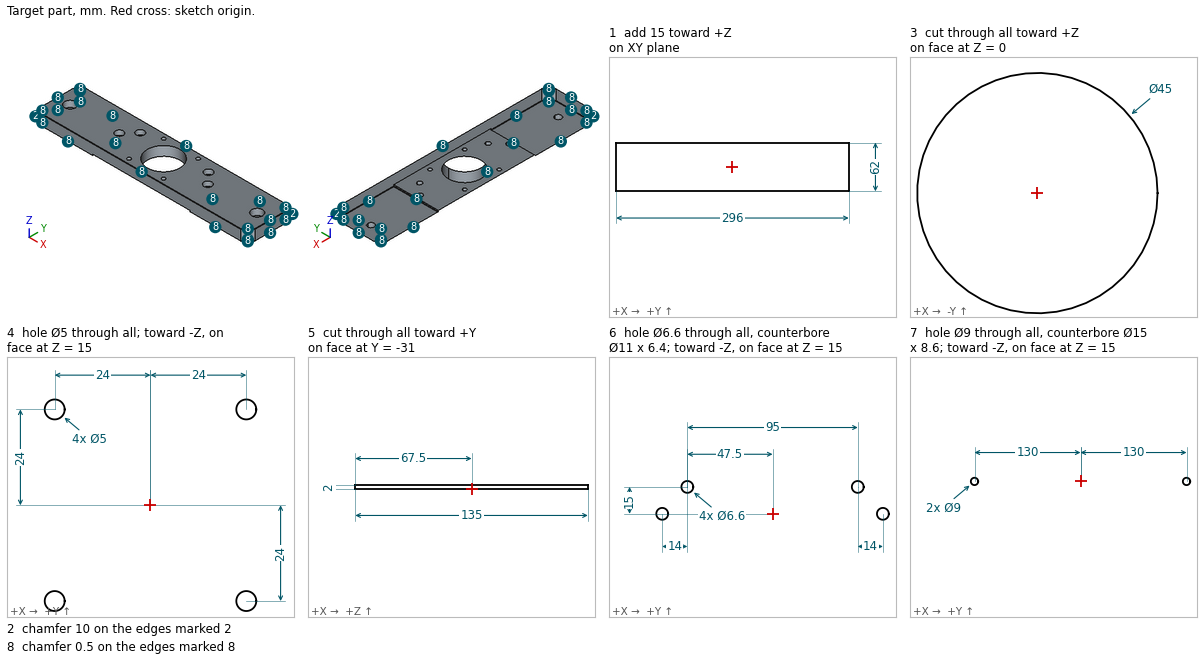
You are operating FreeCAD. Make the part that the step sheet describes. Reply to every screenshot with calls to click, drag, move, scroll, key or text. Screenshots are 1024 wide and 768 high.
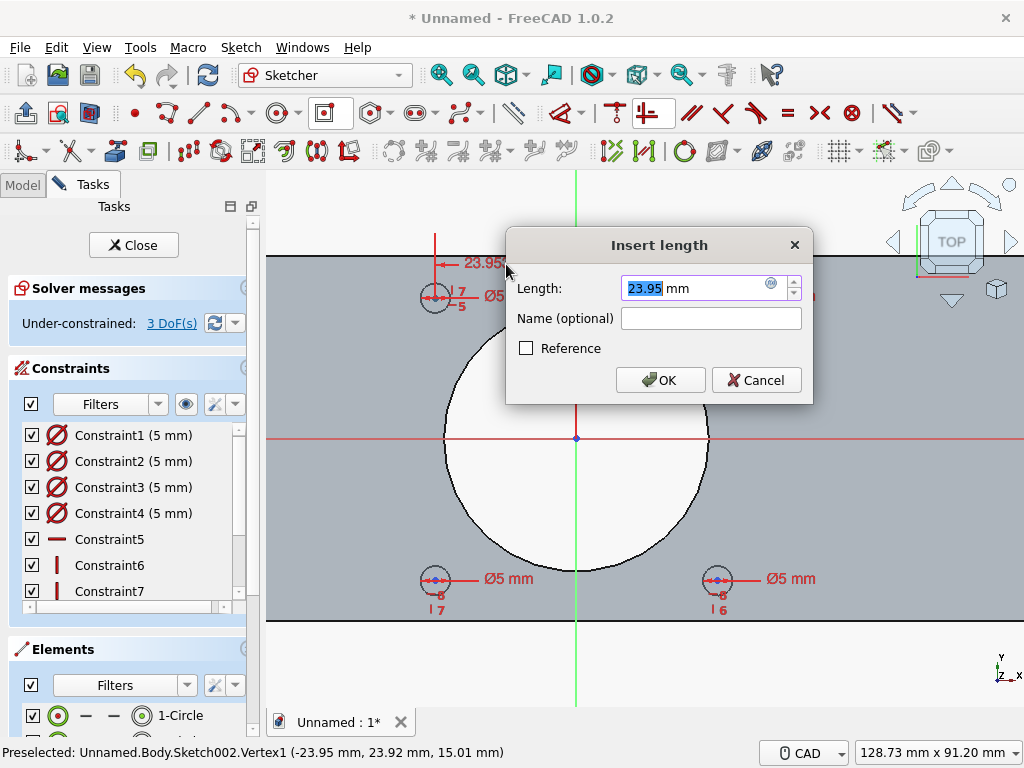
text(24)
key(Return)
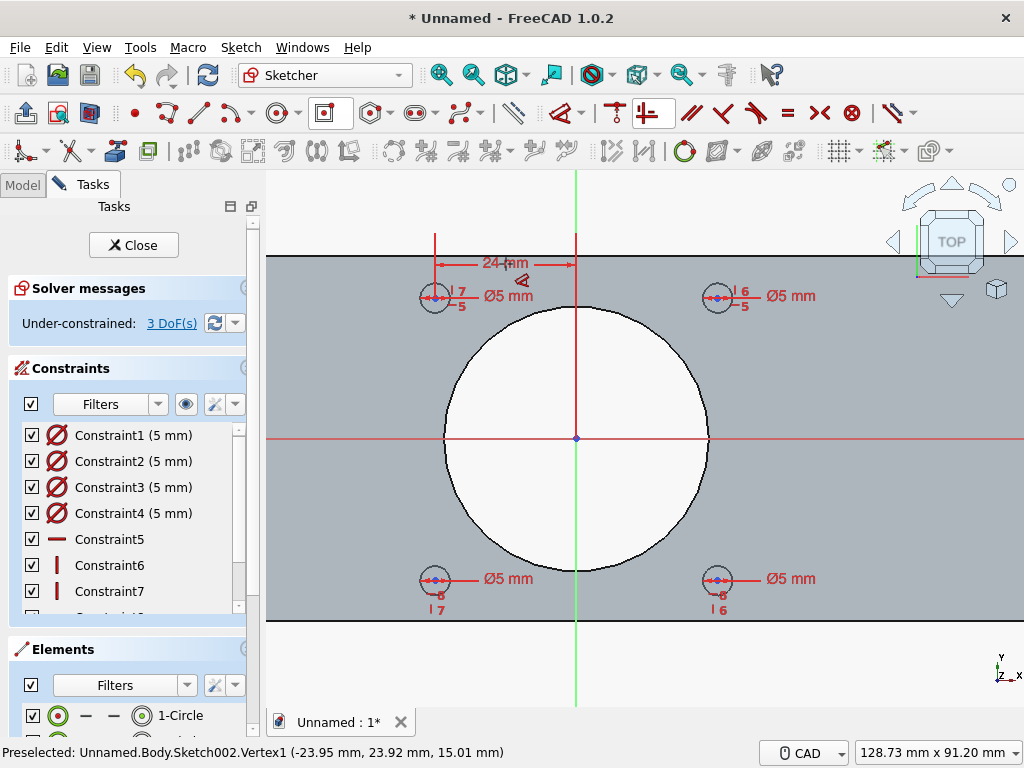
click(435, 298)
click(401, 369)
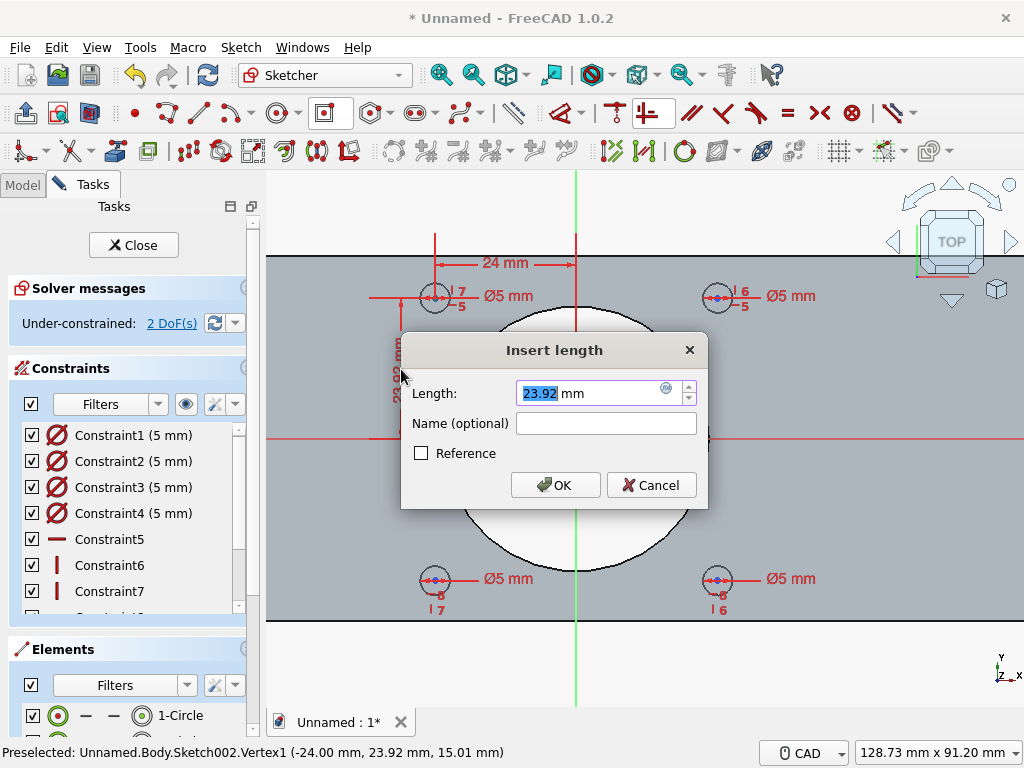
text(24)
key(Return)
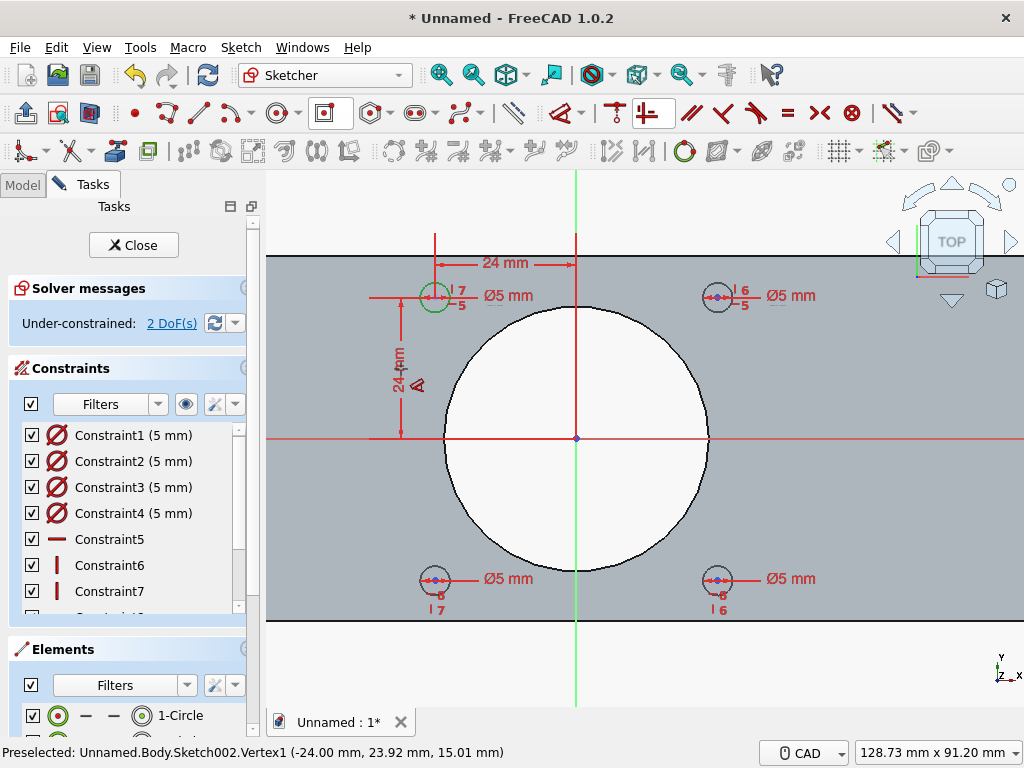
click(718, 298)
click(647, 264)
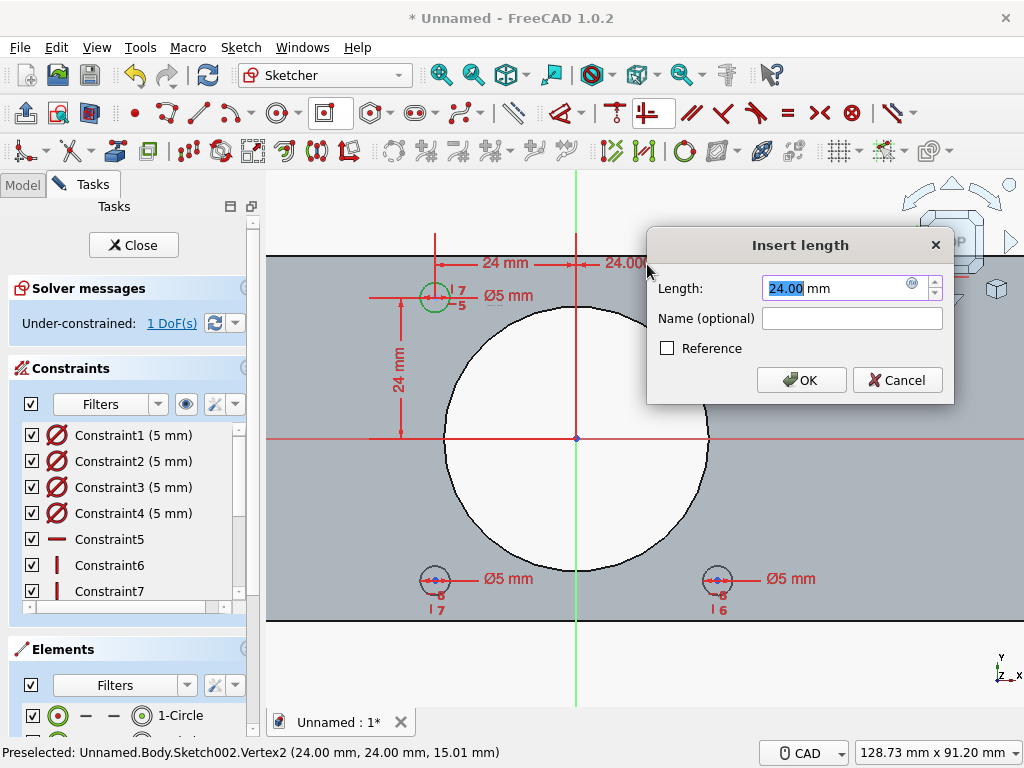
text(24)
key(Return)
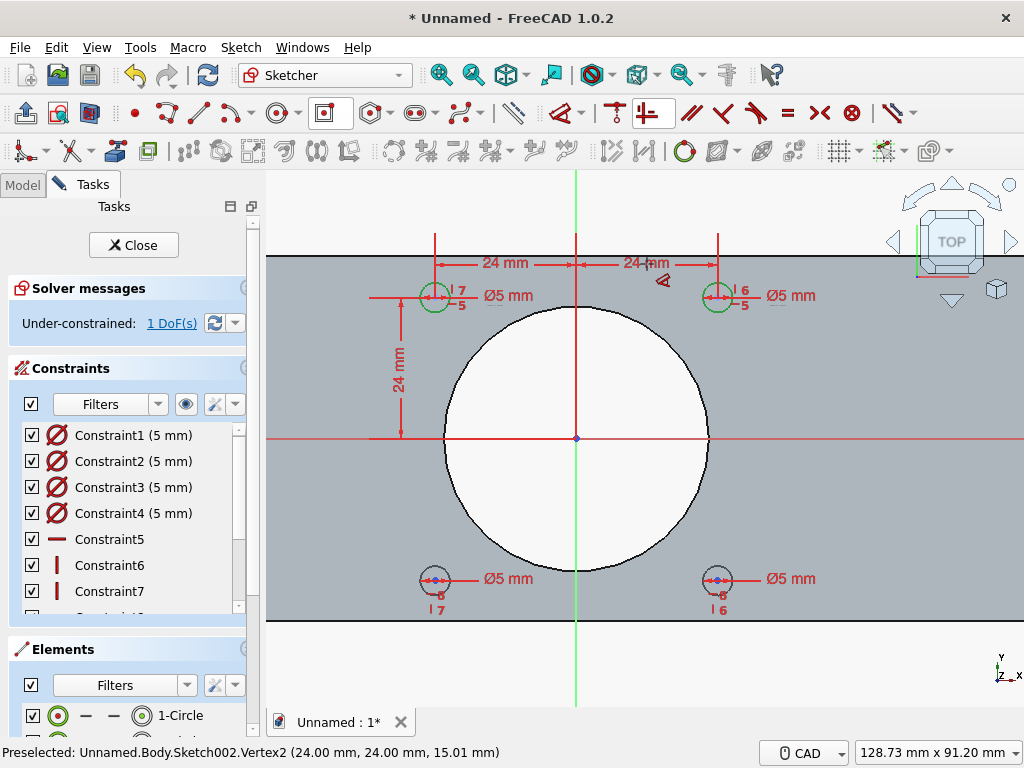
click(718, 581)
click(752, 510)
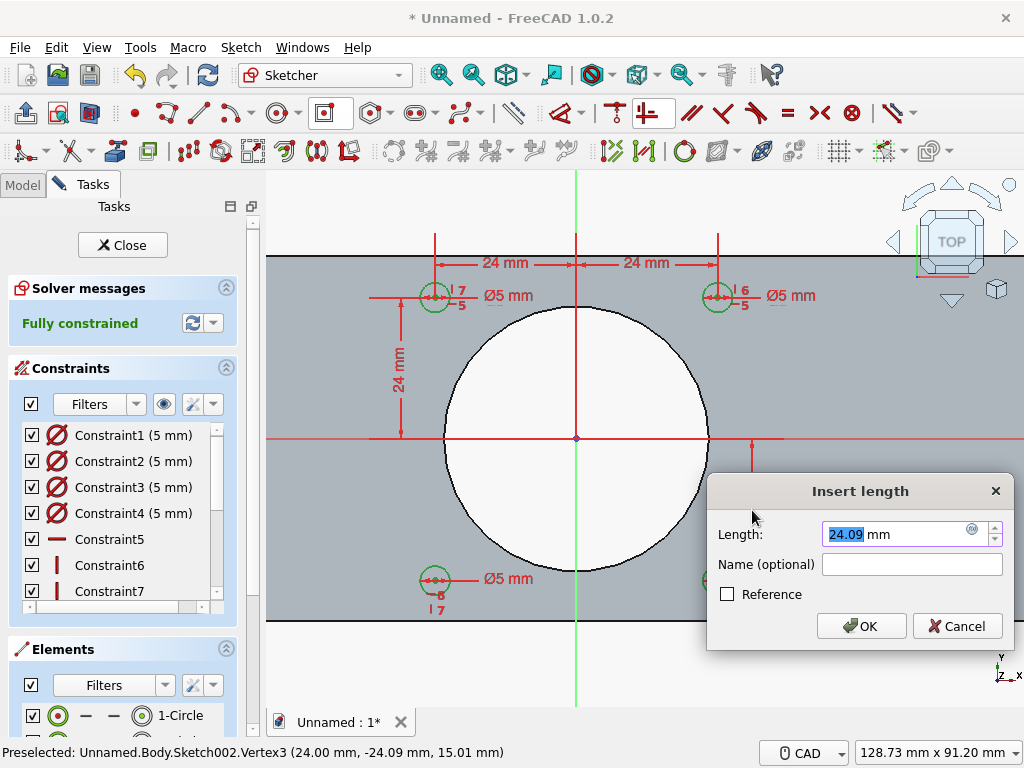
text(24)
key(Return)
key(Escape)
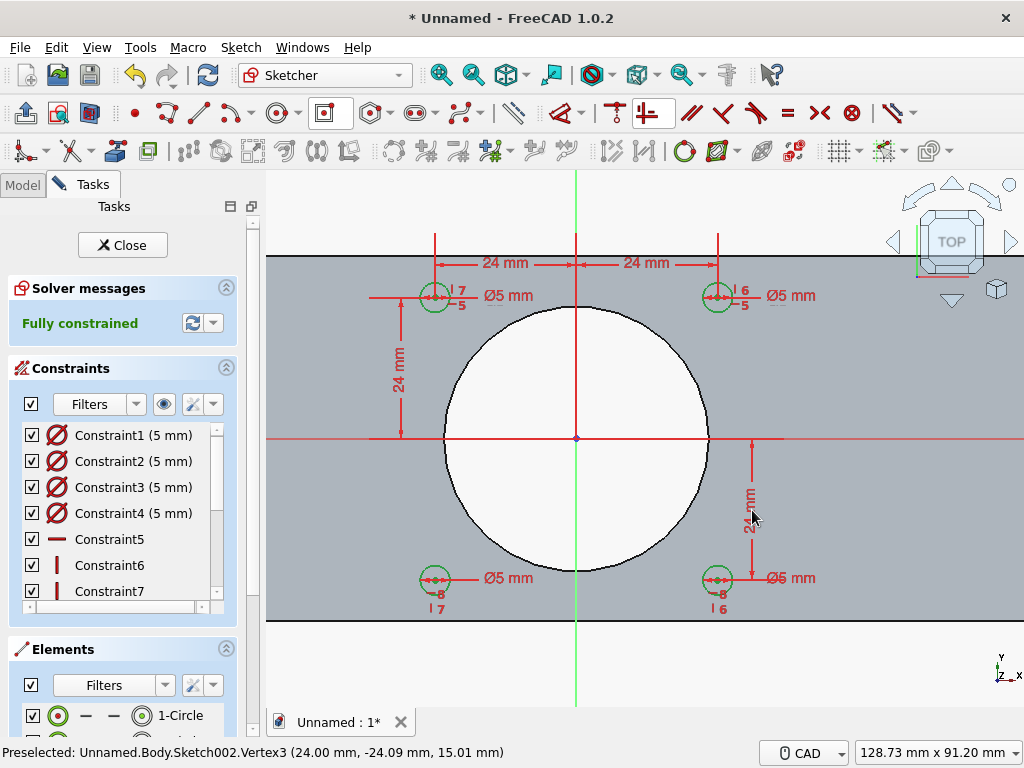
click(123, 245)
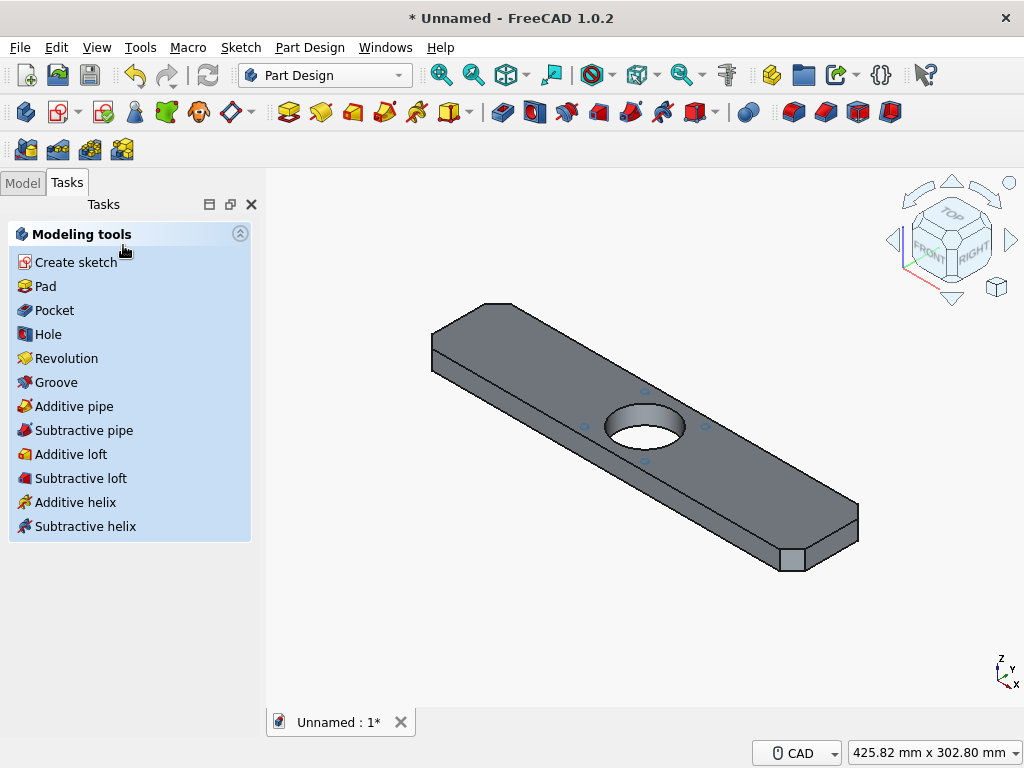
click(536, 112)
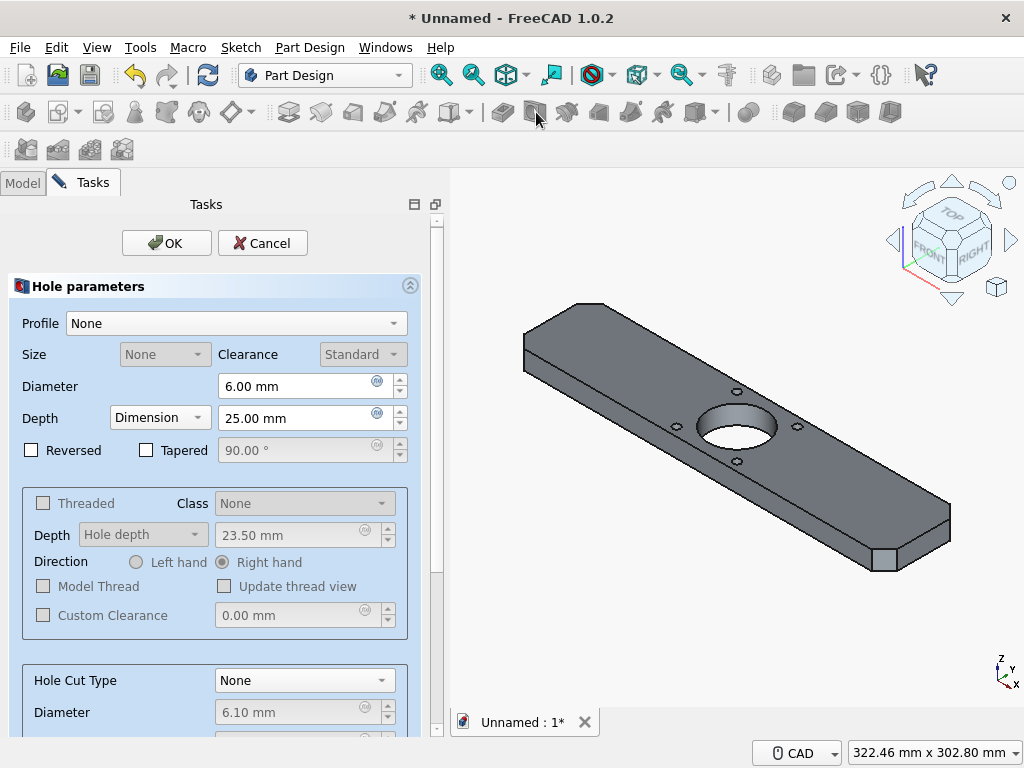
triple_click(305, 386)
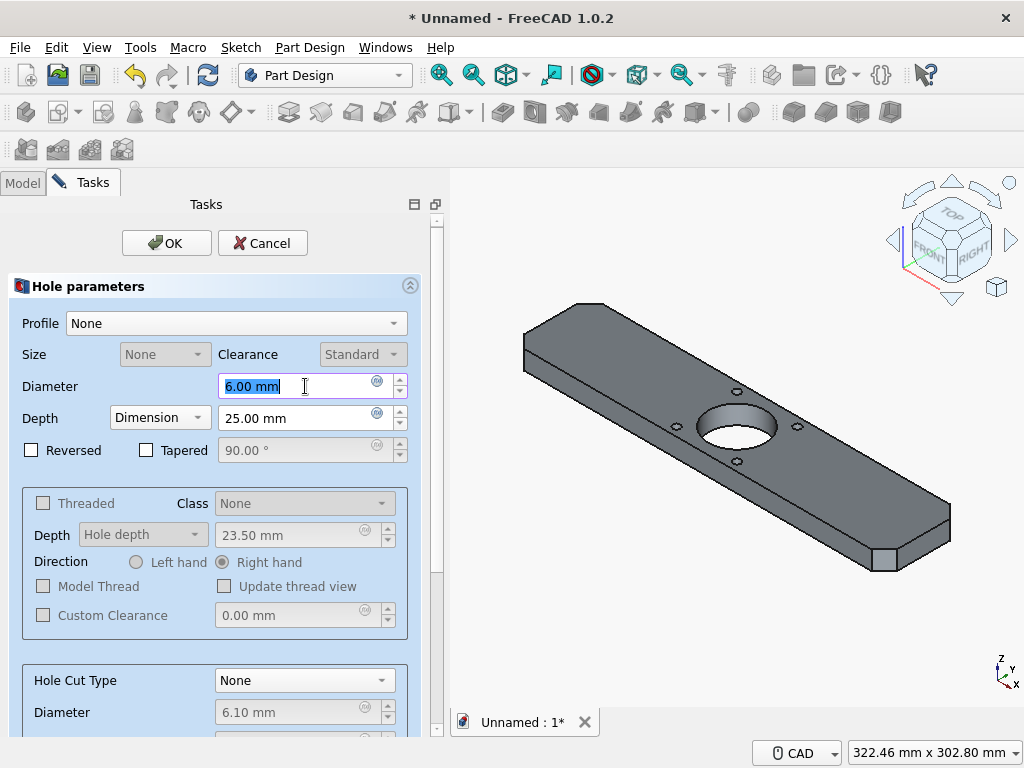
text(5)
key(Tab)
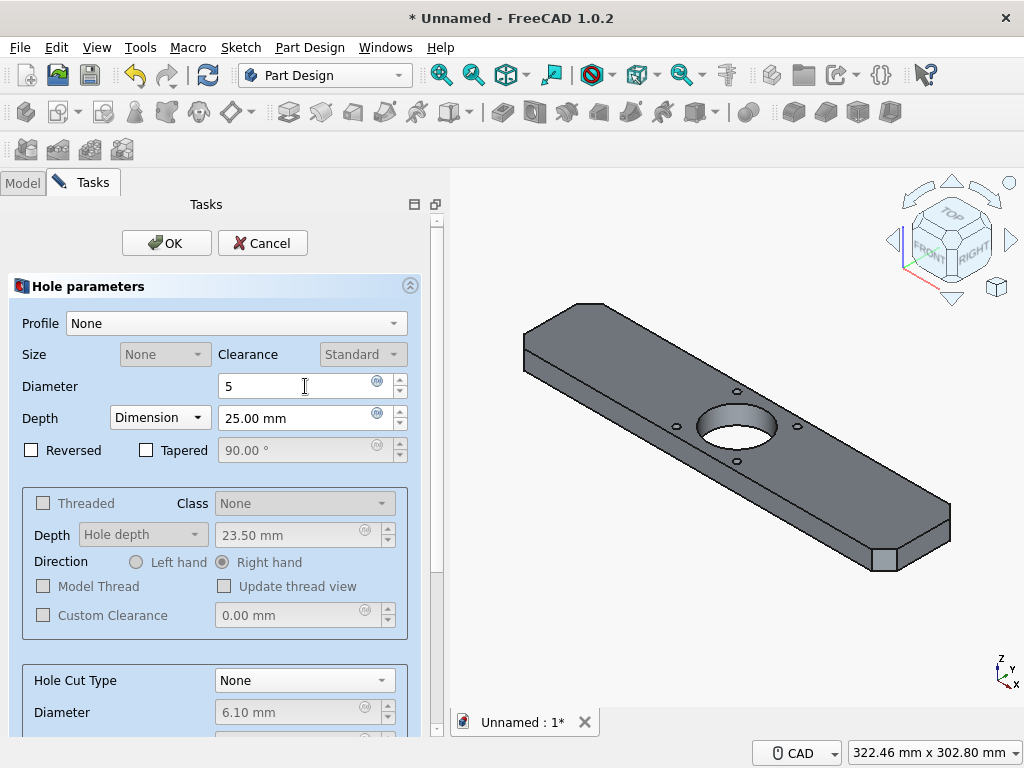
click(161, 418)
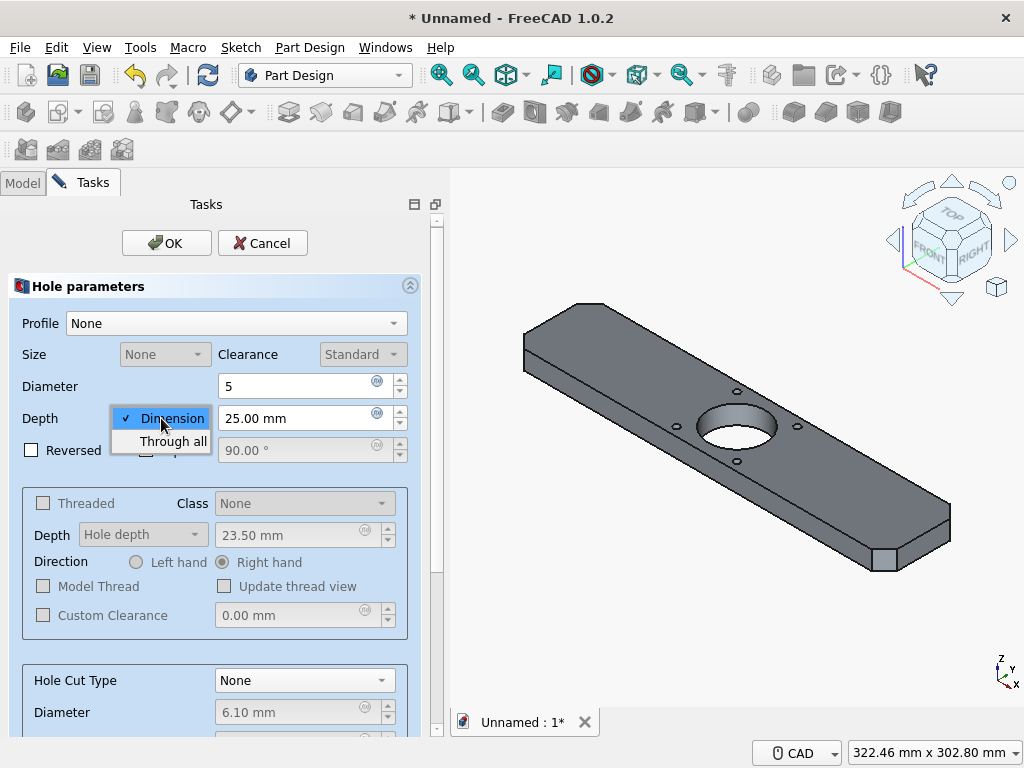
click(160, 442)